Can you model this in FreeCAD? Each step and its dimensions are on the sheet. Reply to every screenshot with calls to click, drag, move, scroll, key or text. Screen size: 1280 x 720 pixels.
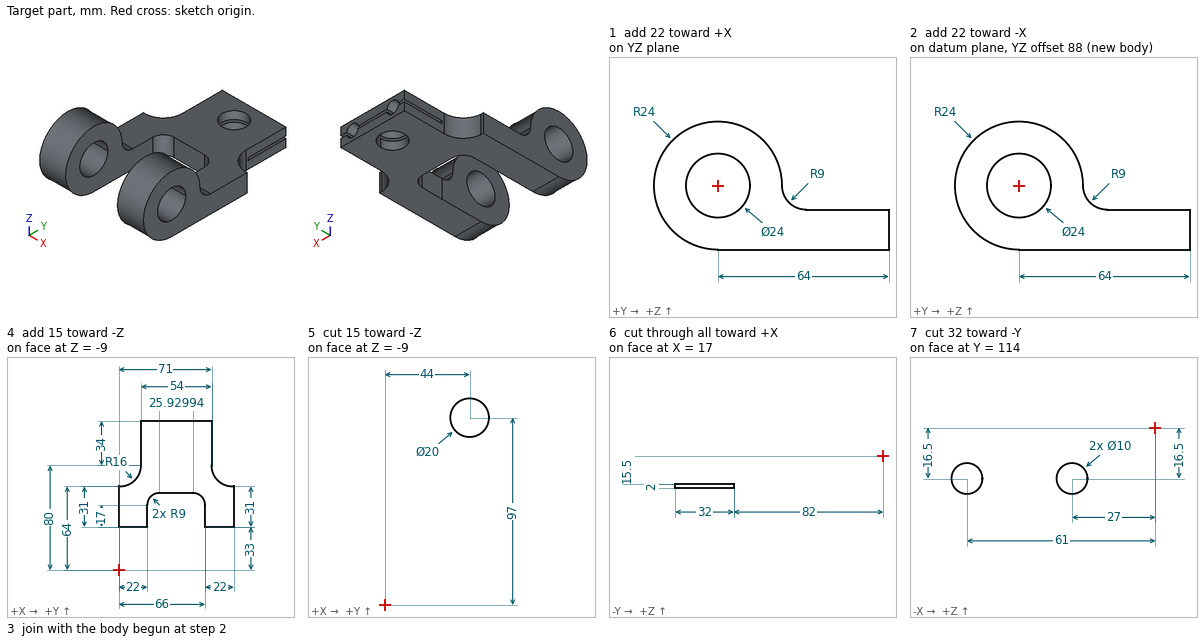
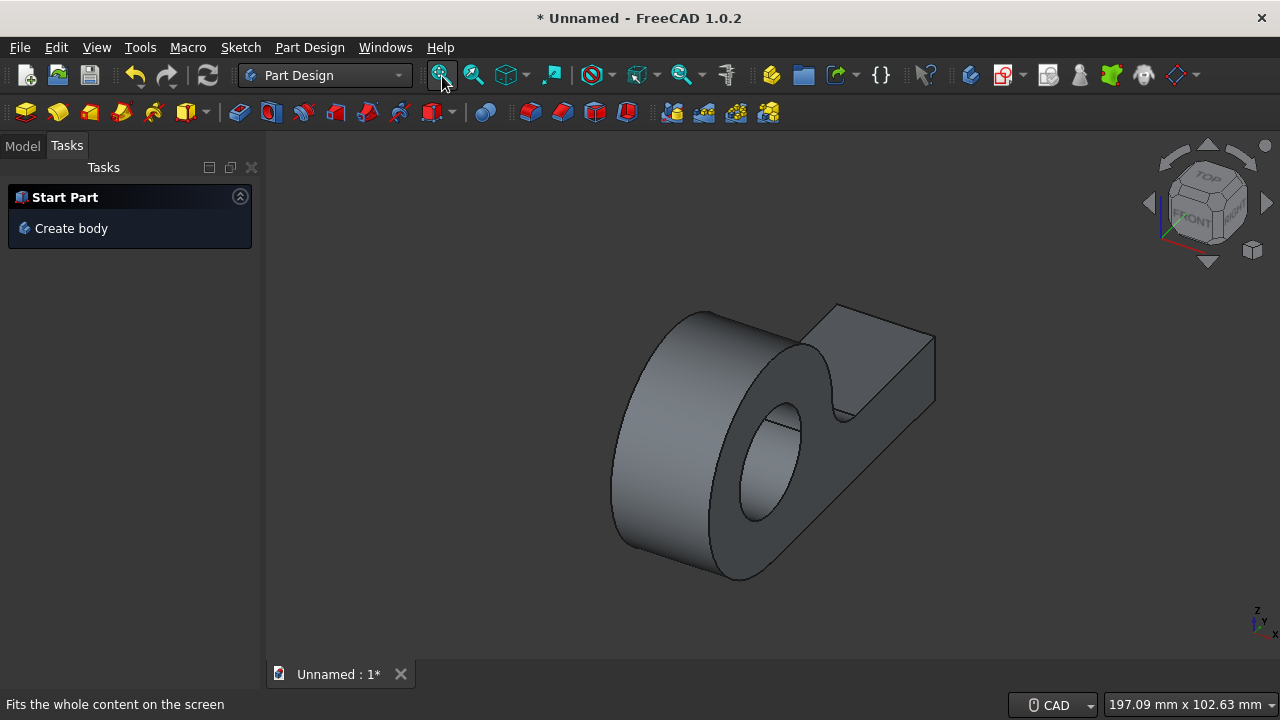
click(972, 76)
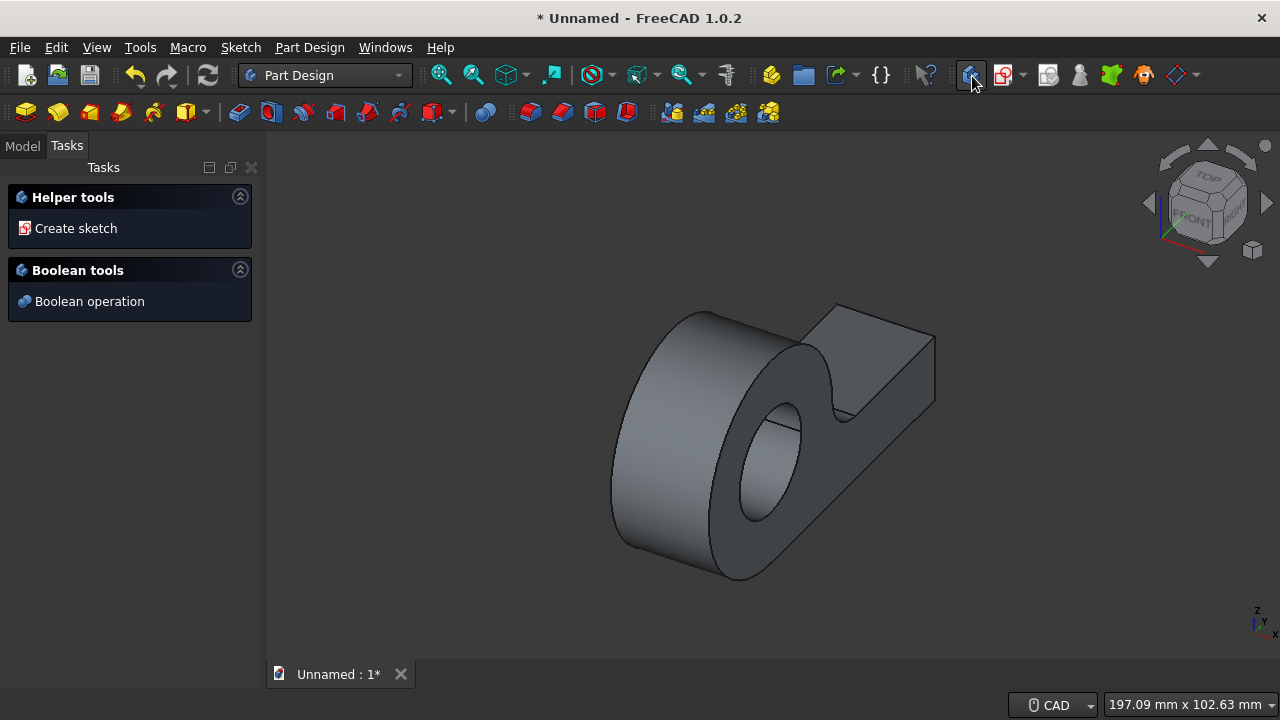
click(23, 145)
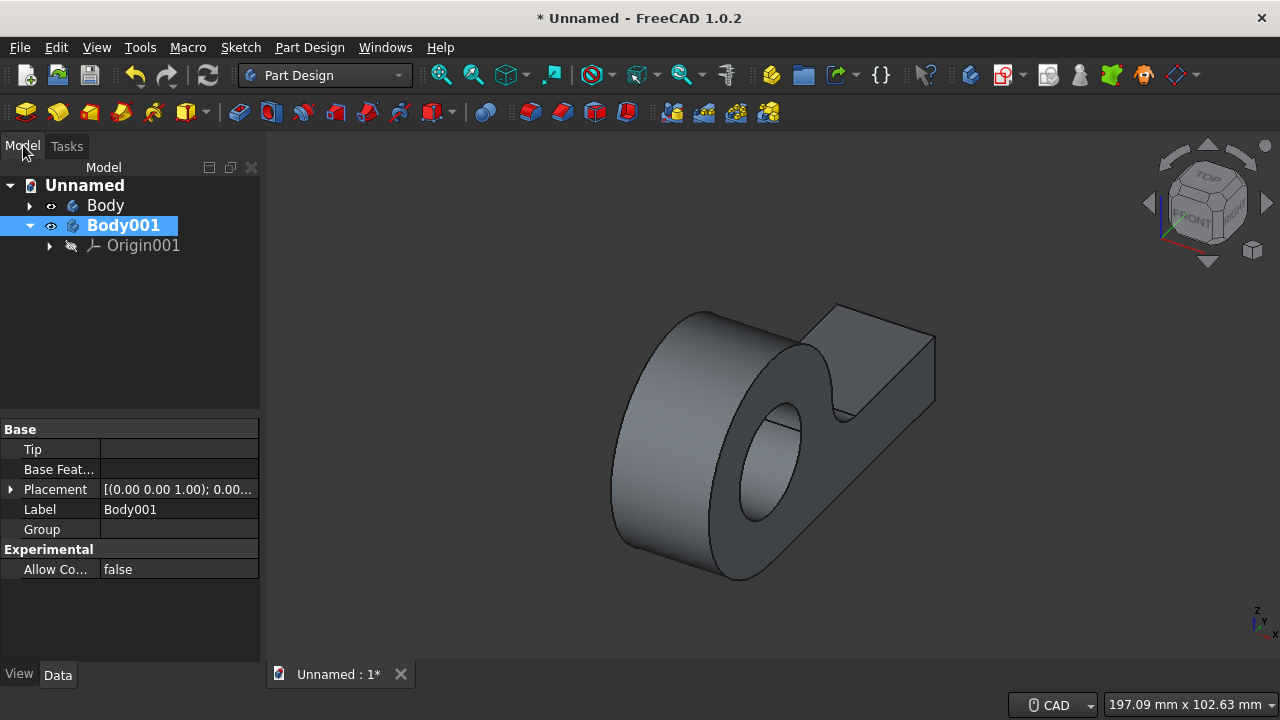
click(50, 246)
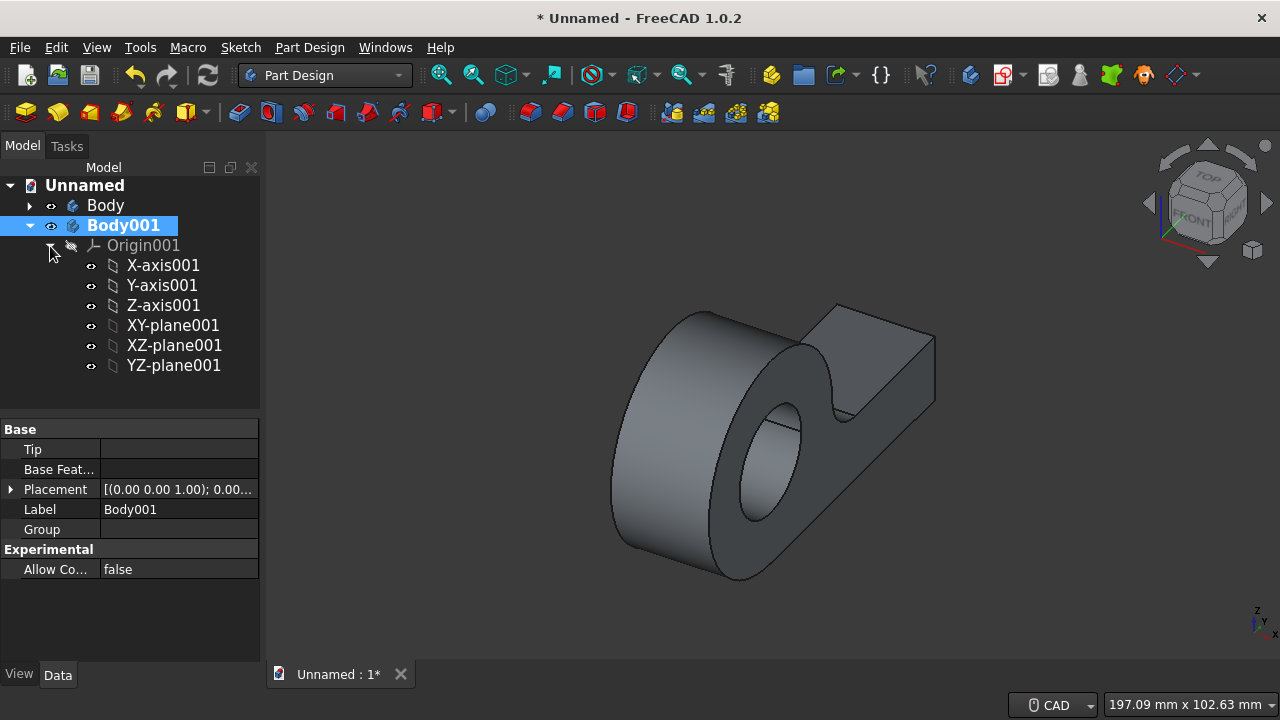
click(136, 366)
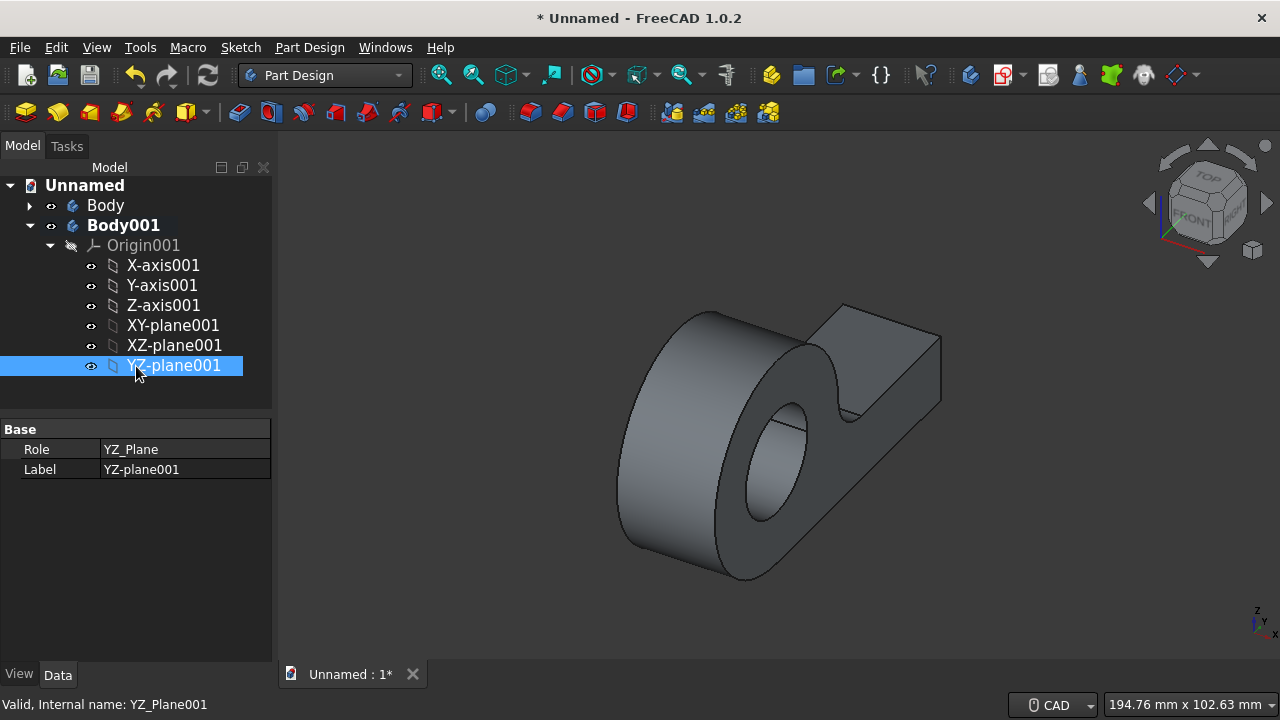
click(1176, 76)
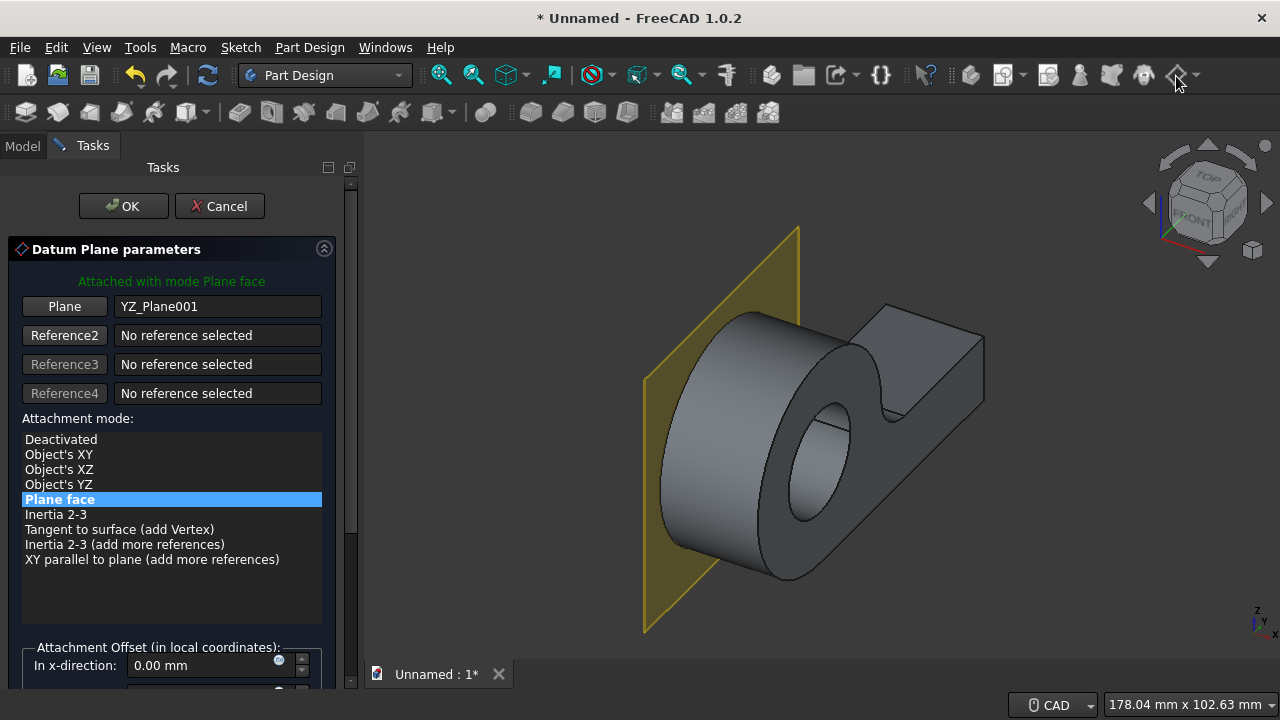
scroll(351, 432, down, 2)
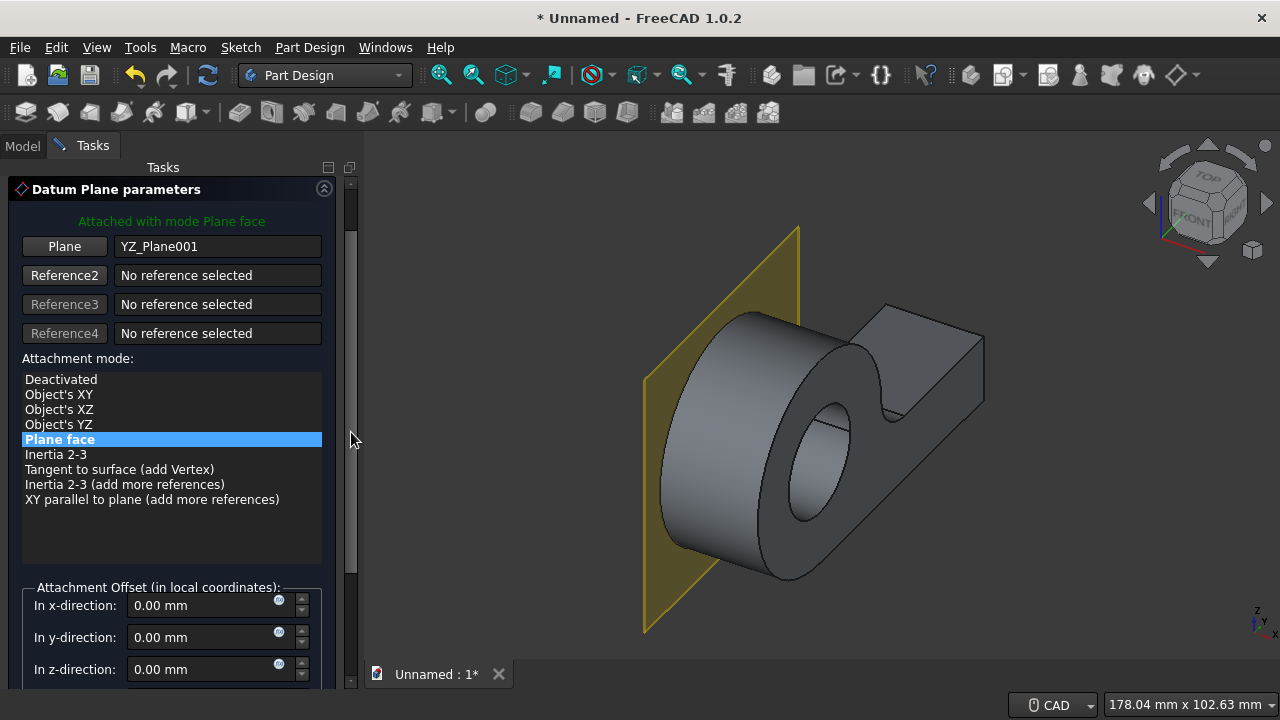
triple_click(210, 609)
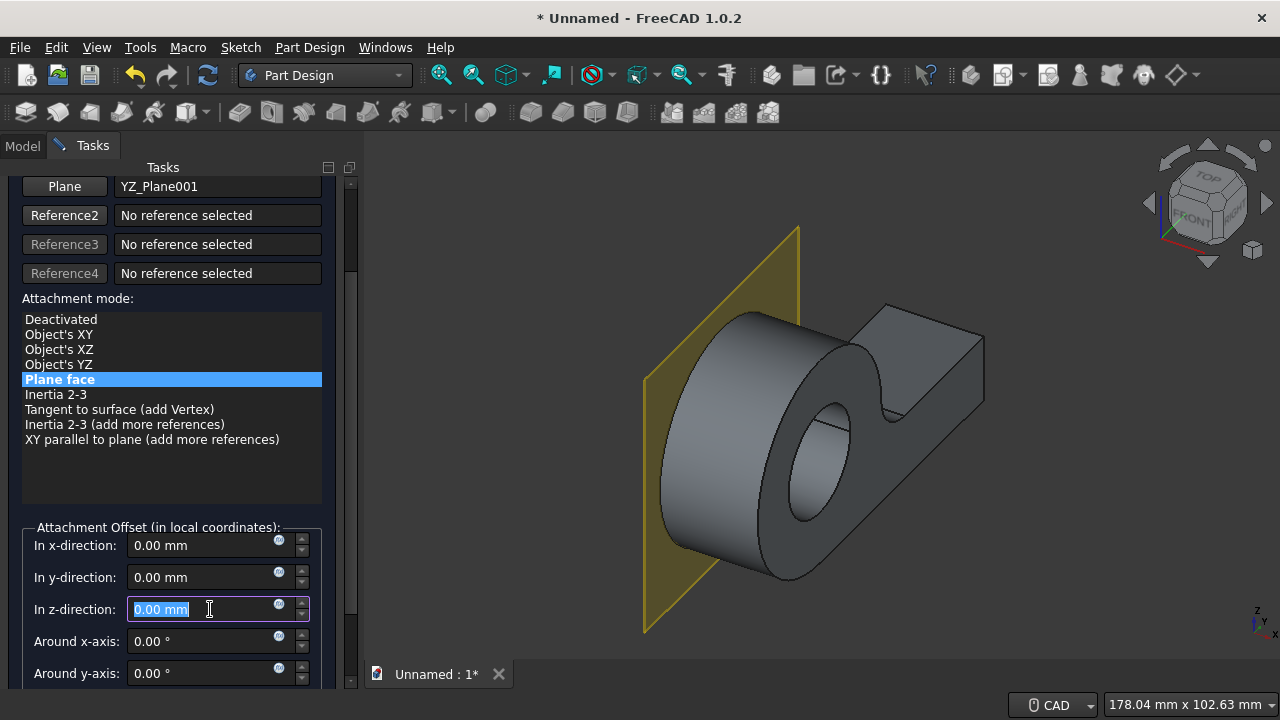
text(88)
key(Tab)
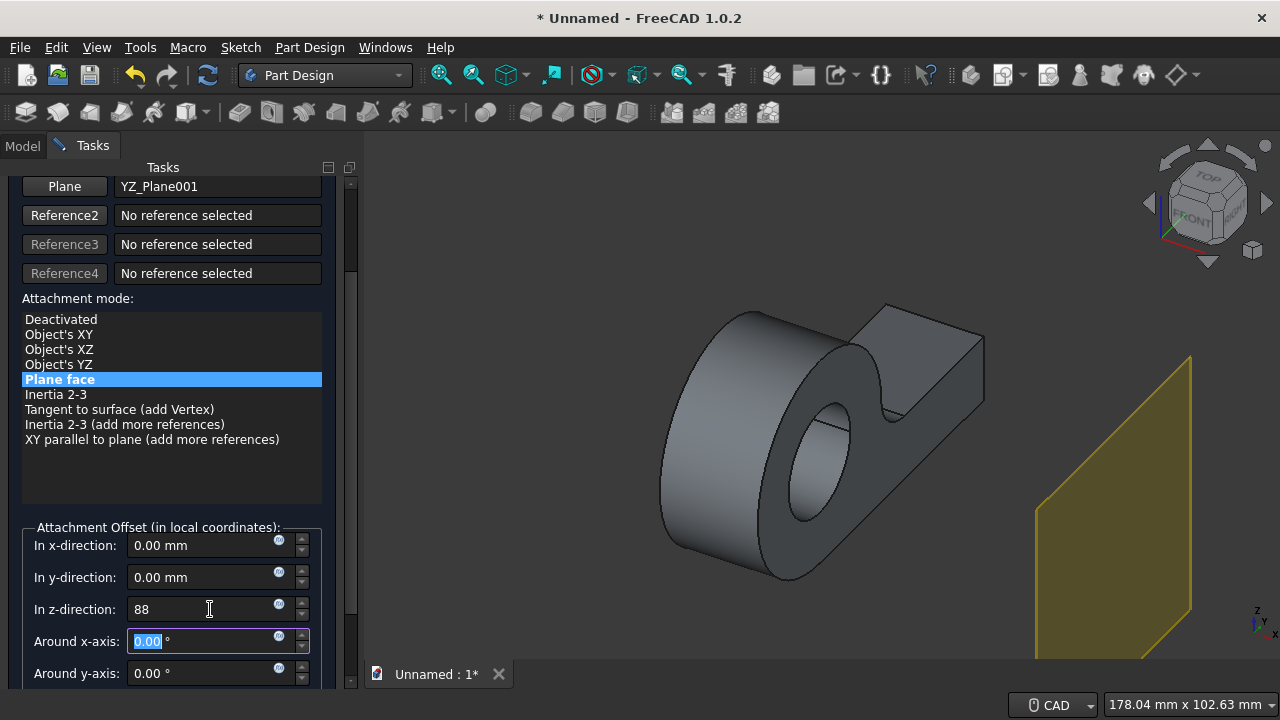
scroll(351, 432, up, 3)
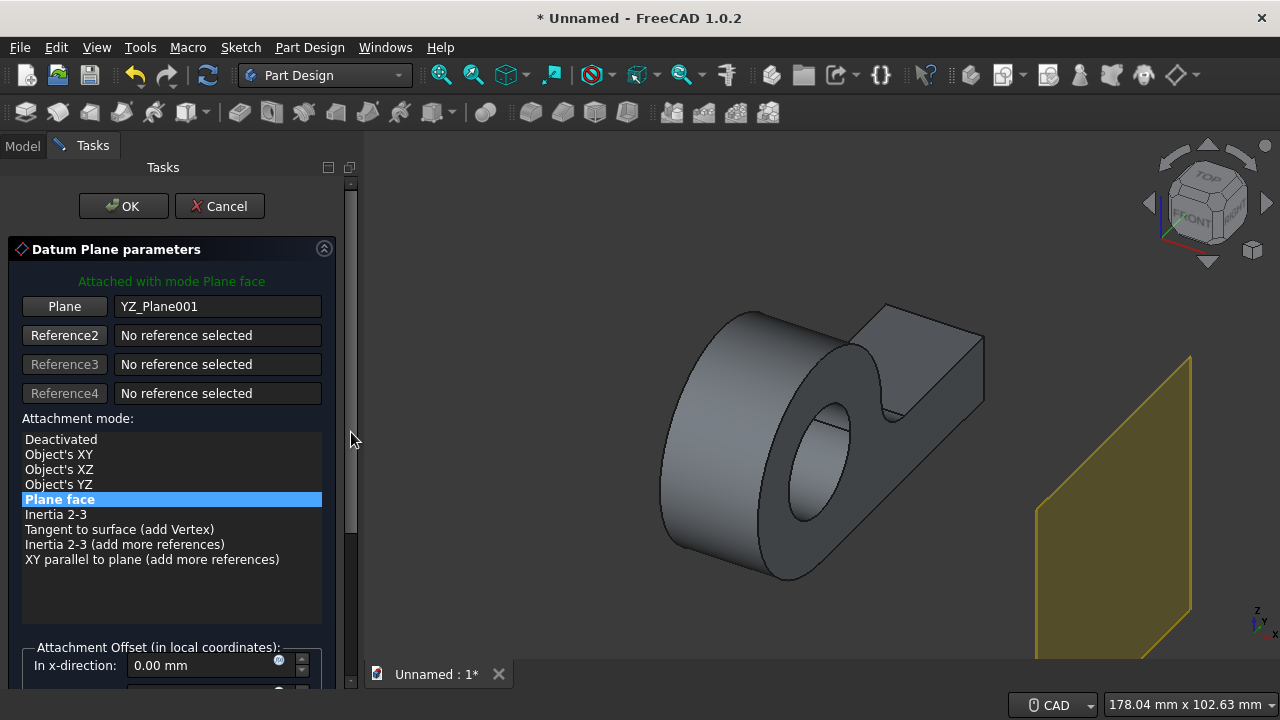
click(124, 206)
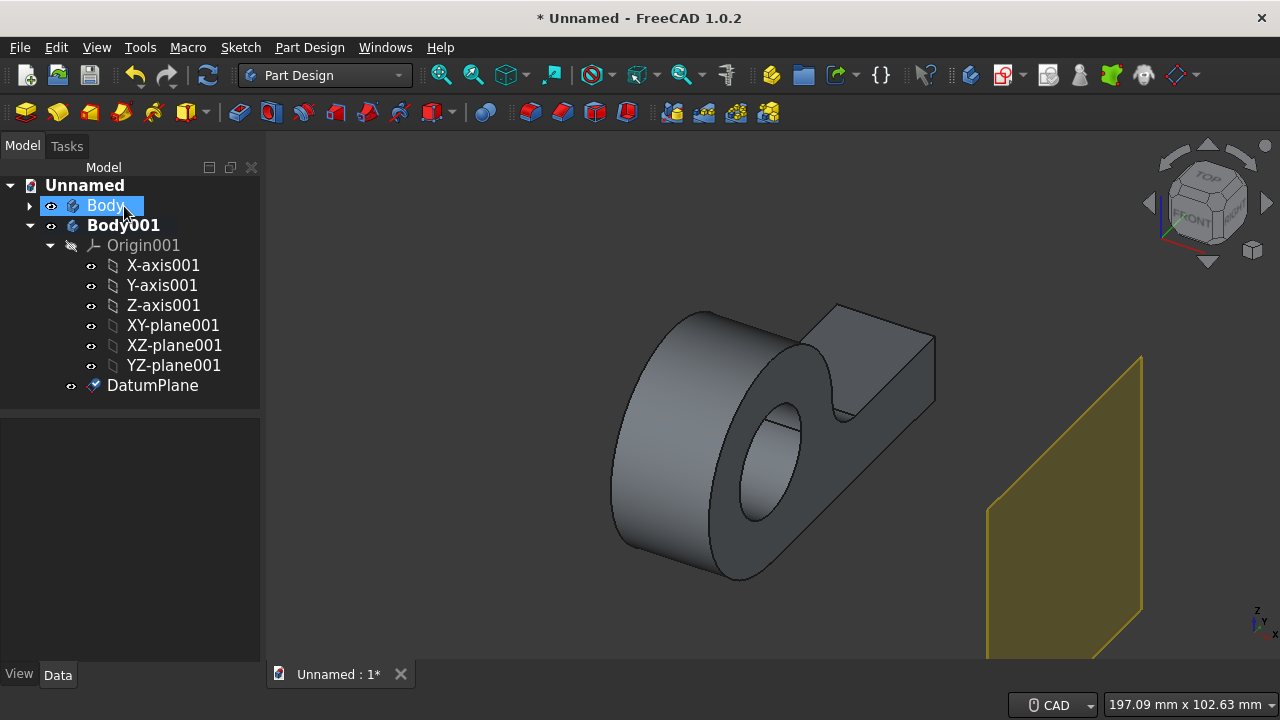
click(116, 386)